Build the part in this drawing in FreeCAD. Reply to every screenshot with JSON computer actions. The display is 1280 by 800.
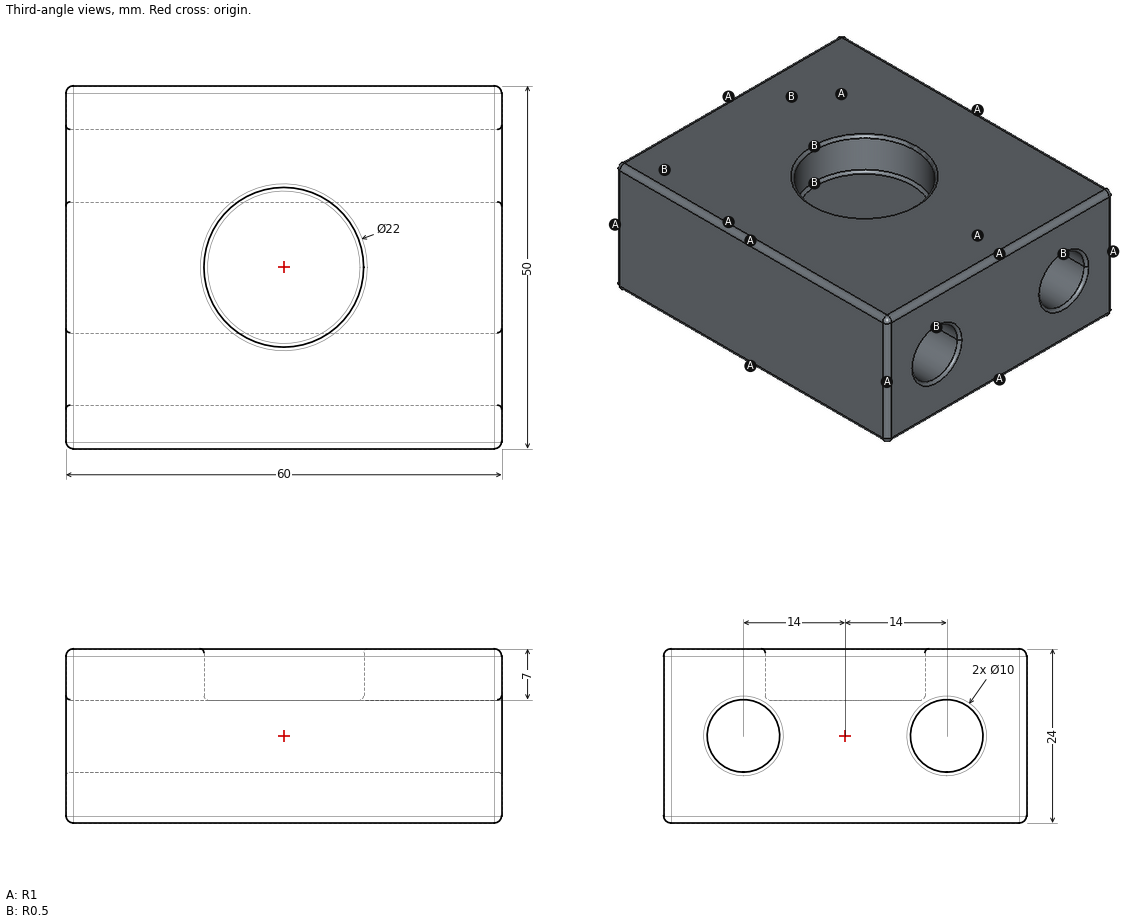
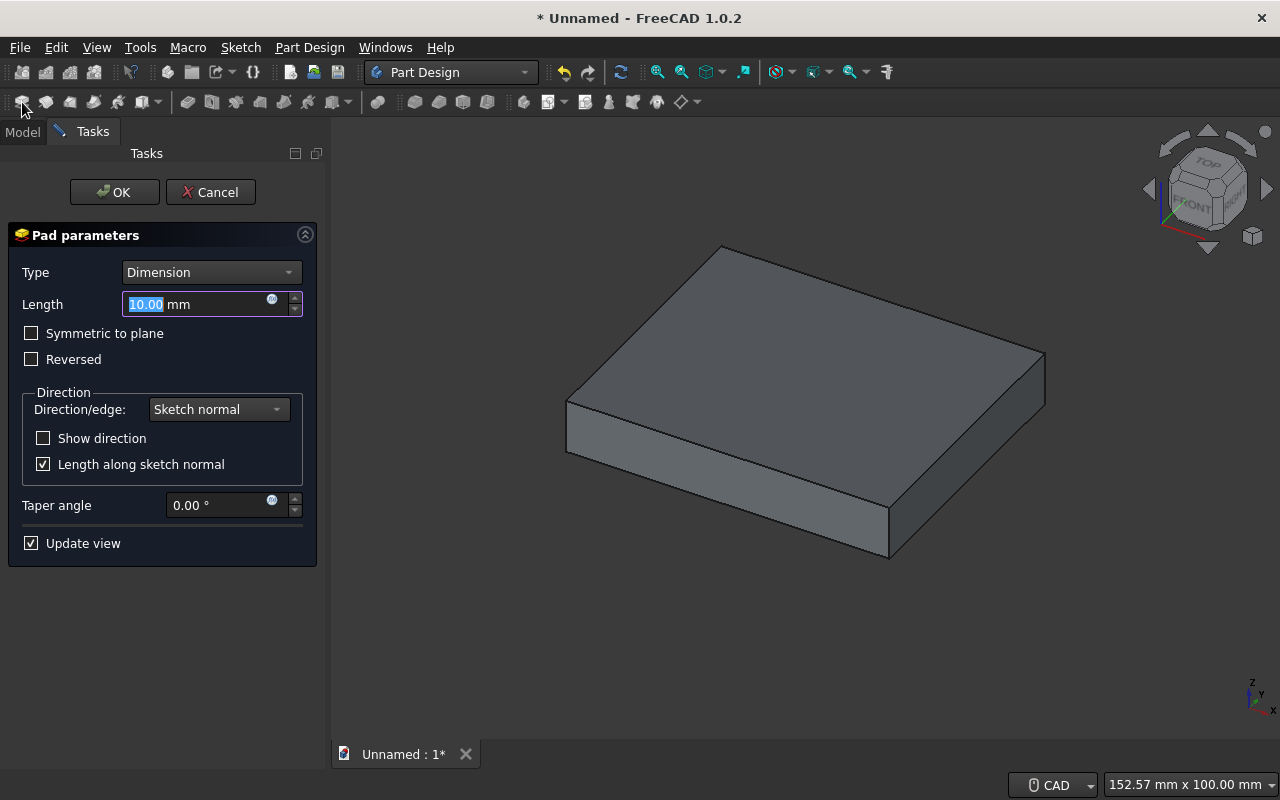
{"action": "type", "text": "24"}
{"action": "key", "text": "Tab"}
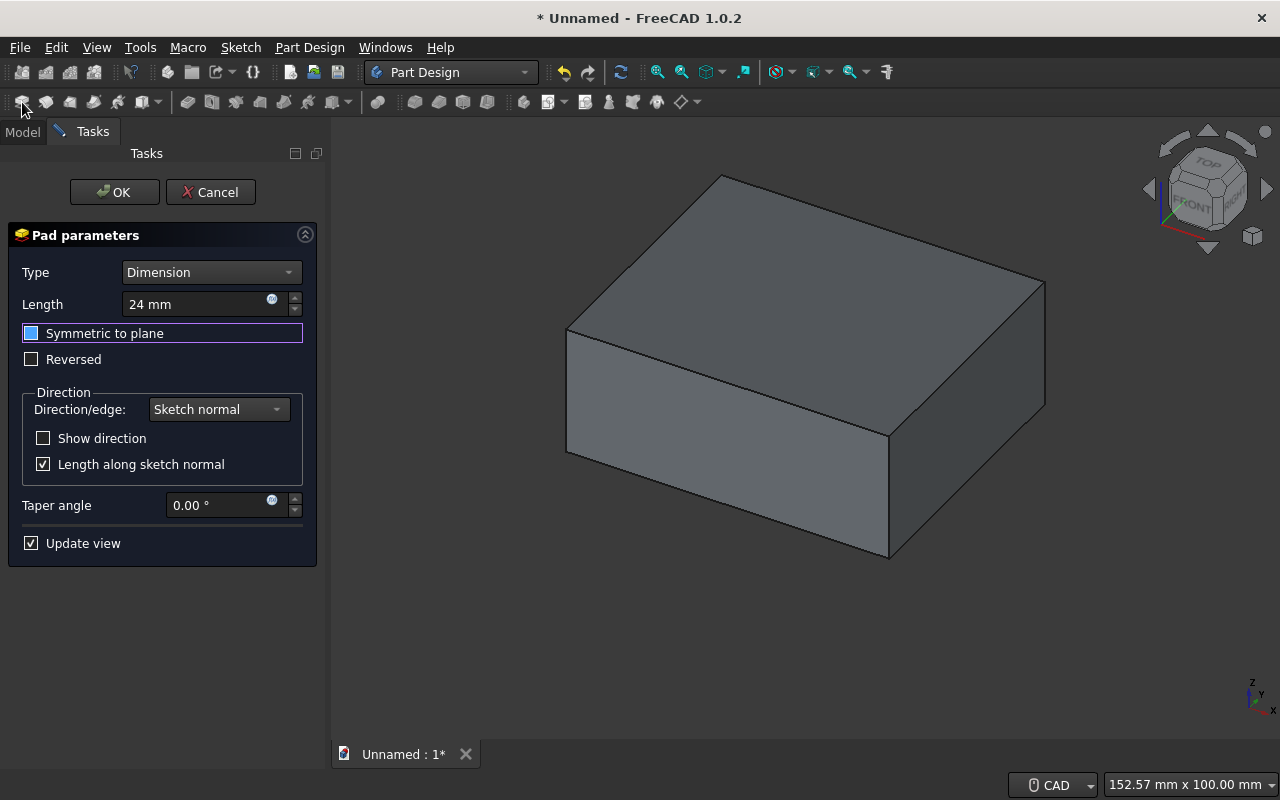
{"action": "left_click", "coordinate": [30, 333]}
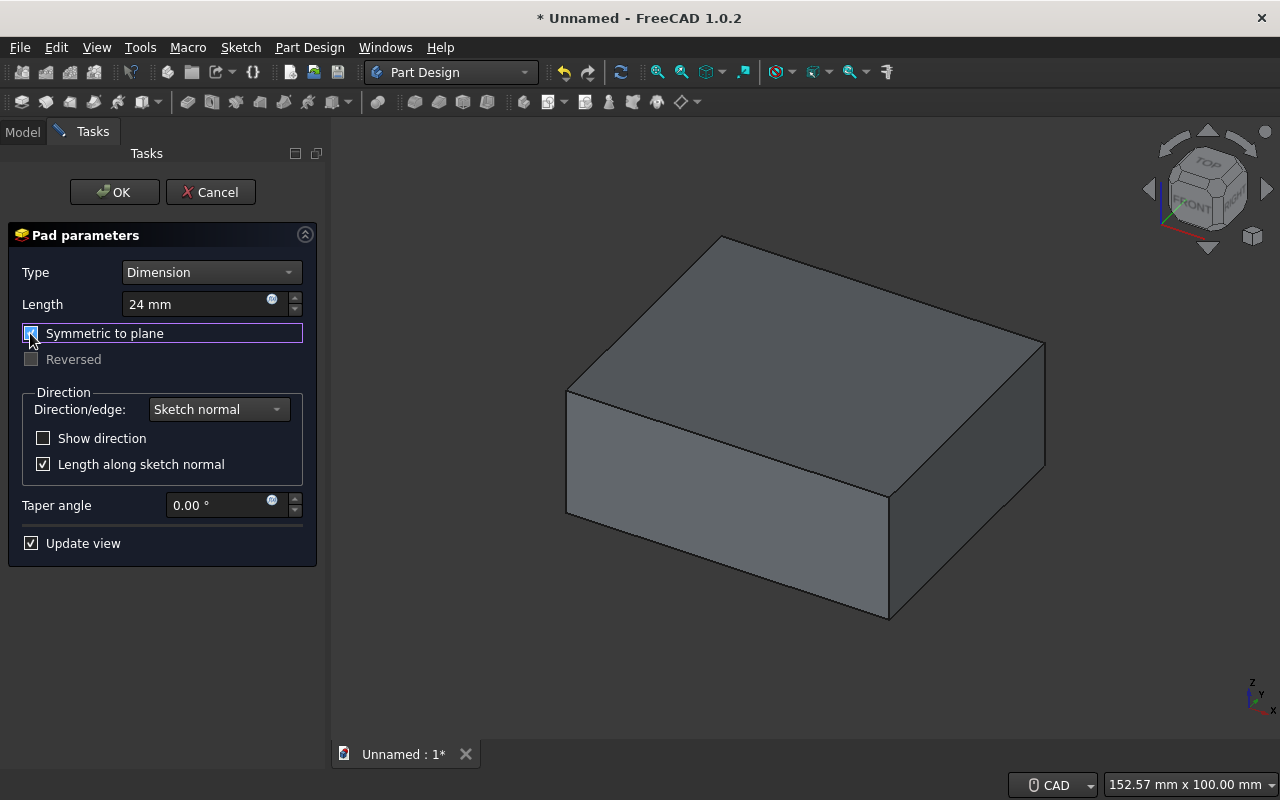
{"action": "left_click", "coordinate": [115, 192]}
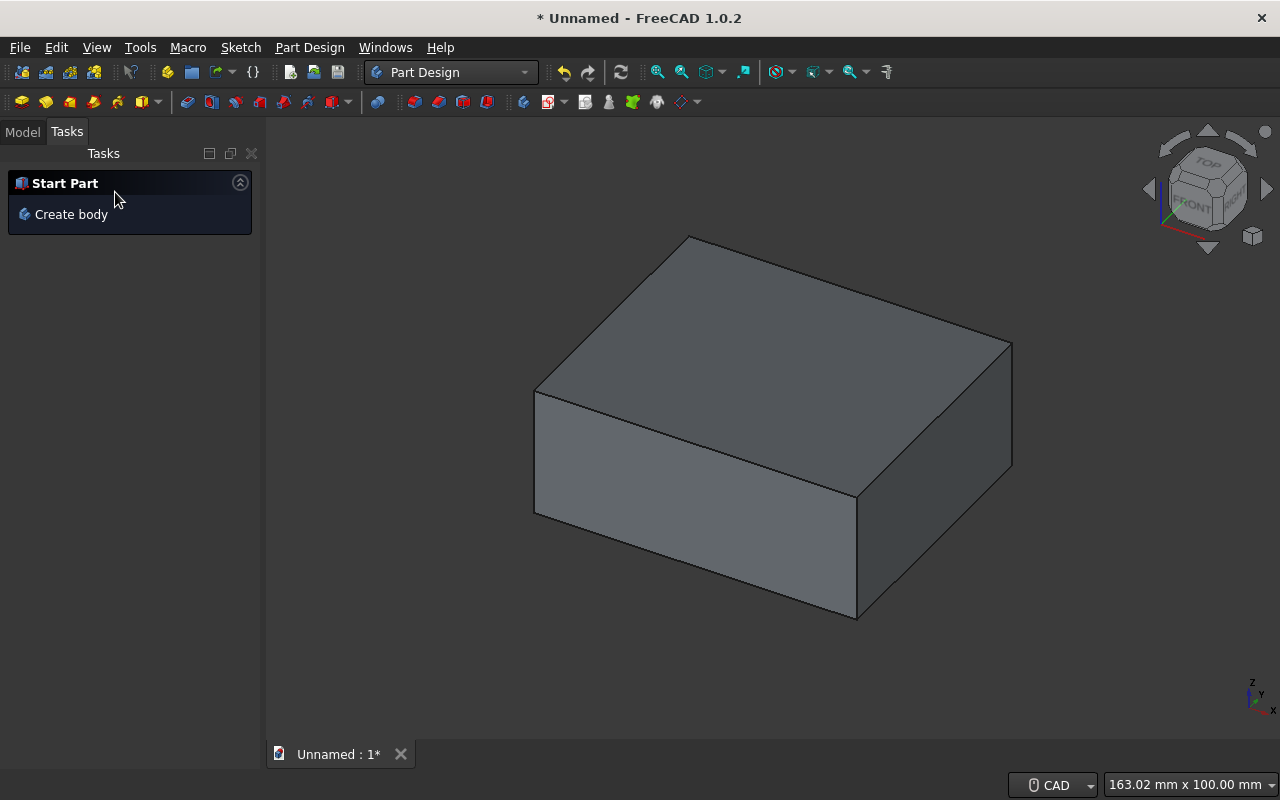
{"action": "left_click", "coordinate": [773, 366]}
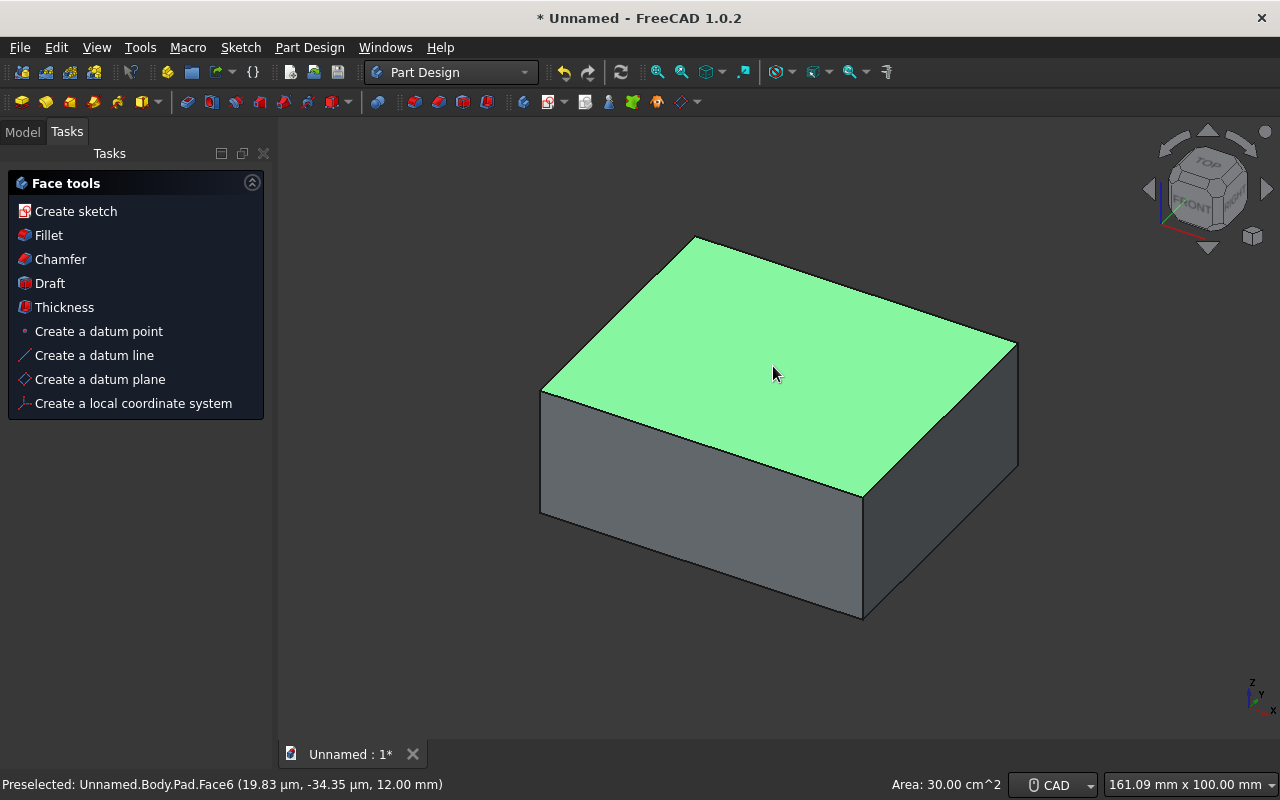
{"action": "left_click", "coordinate": [548, 102]}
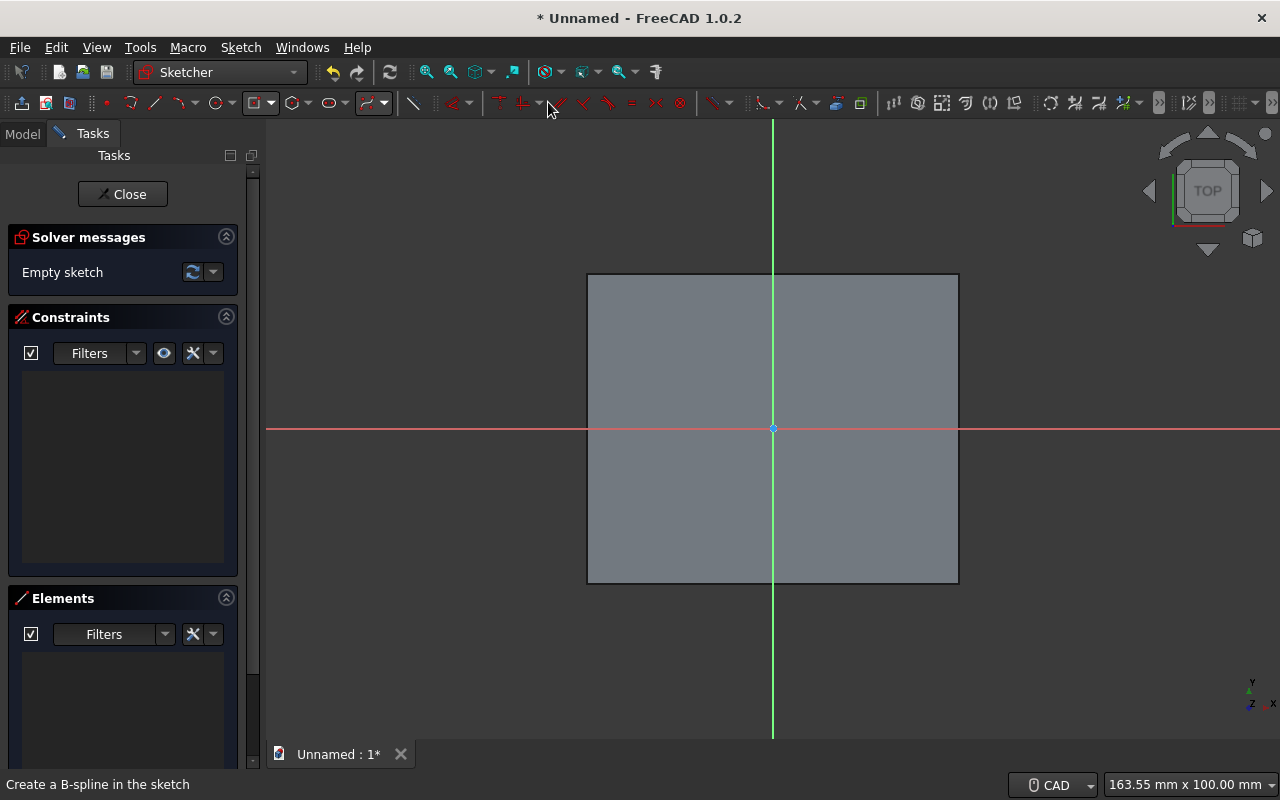
{"action": "scroll", "coordinate": [813, 429], "scroll_direction": "up", "scroll_amount": 5}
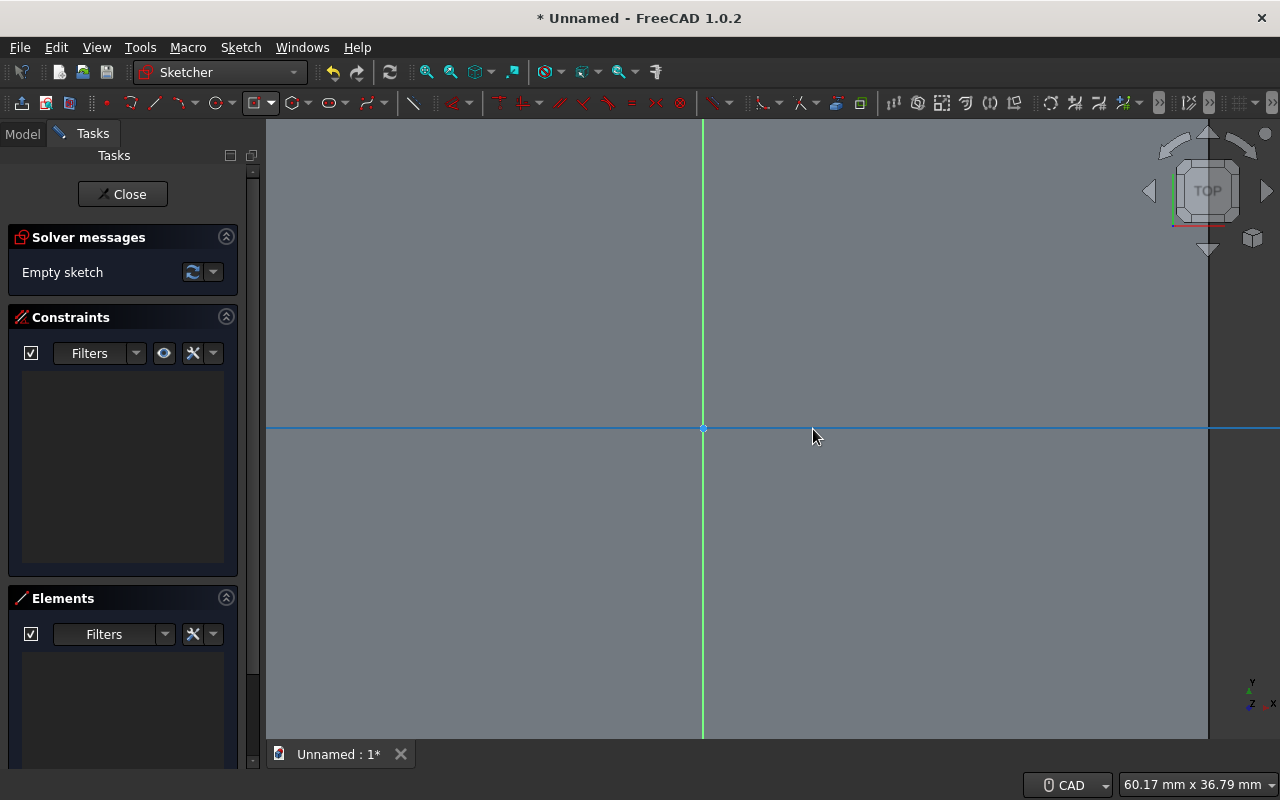
{"action": "left_click", "coordinate": [216, 104]}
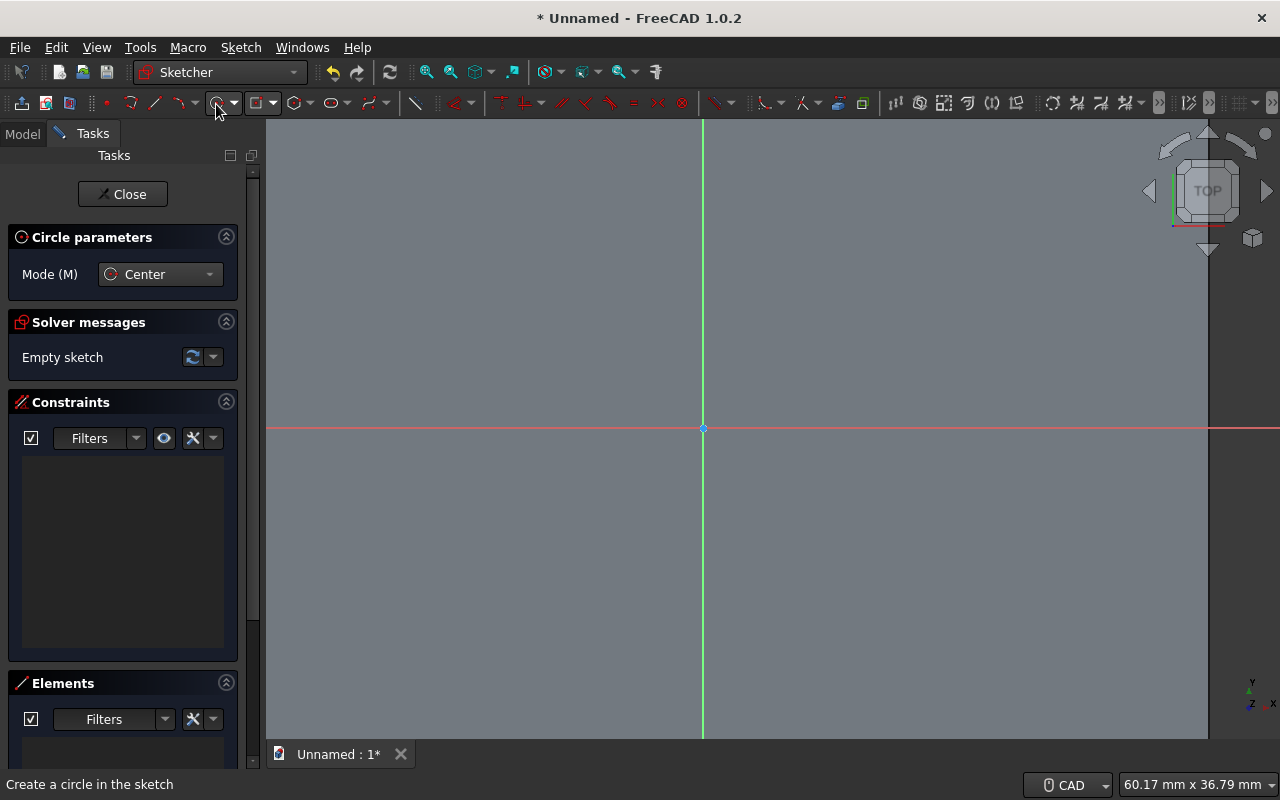
{"action": "left_click", "coordinate": [703, 428]}
{"action": "mouse_move", "coordinate": [834, 297]}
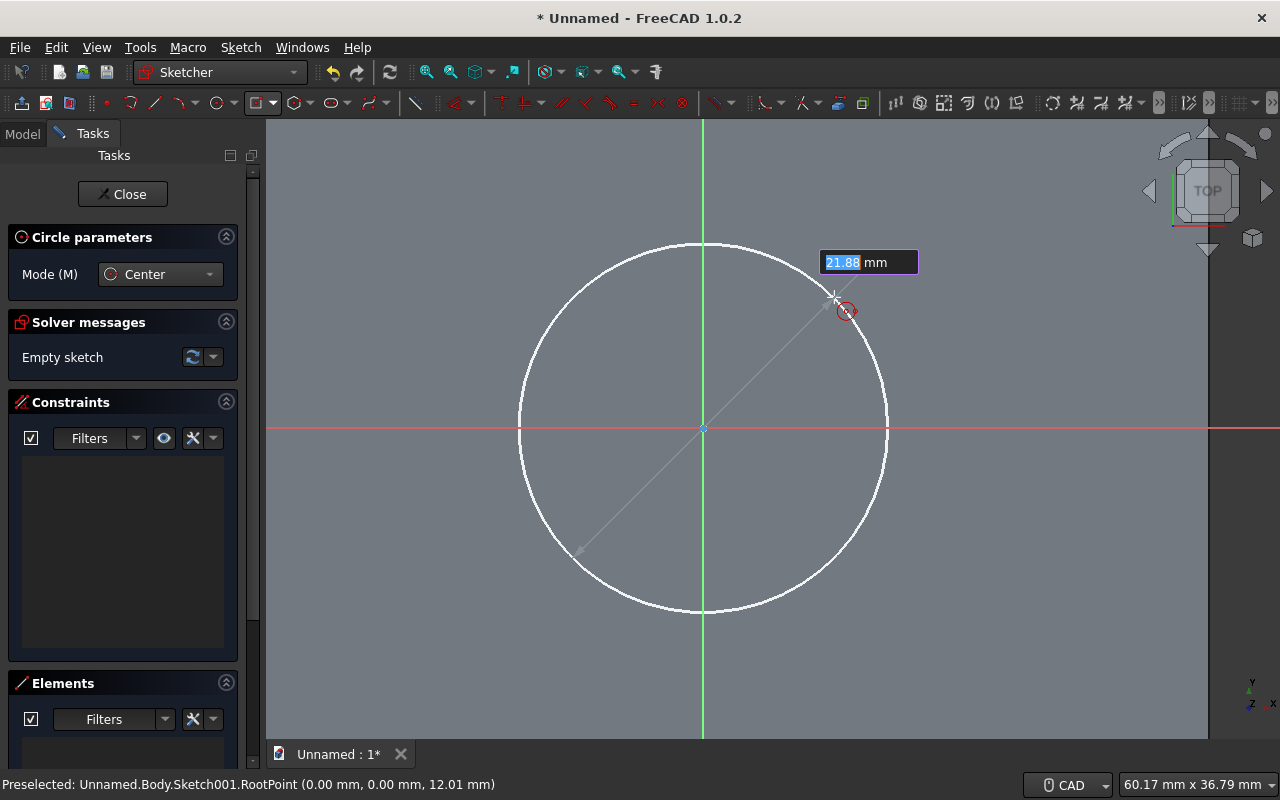
{"action": "type", "text": "22"}
{"action": "key", "text": "Return"}
{"action": "key", "text": "Escape"}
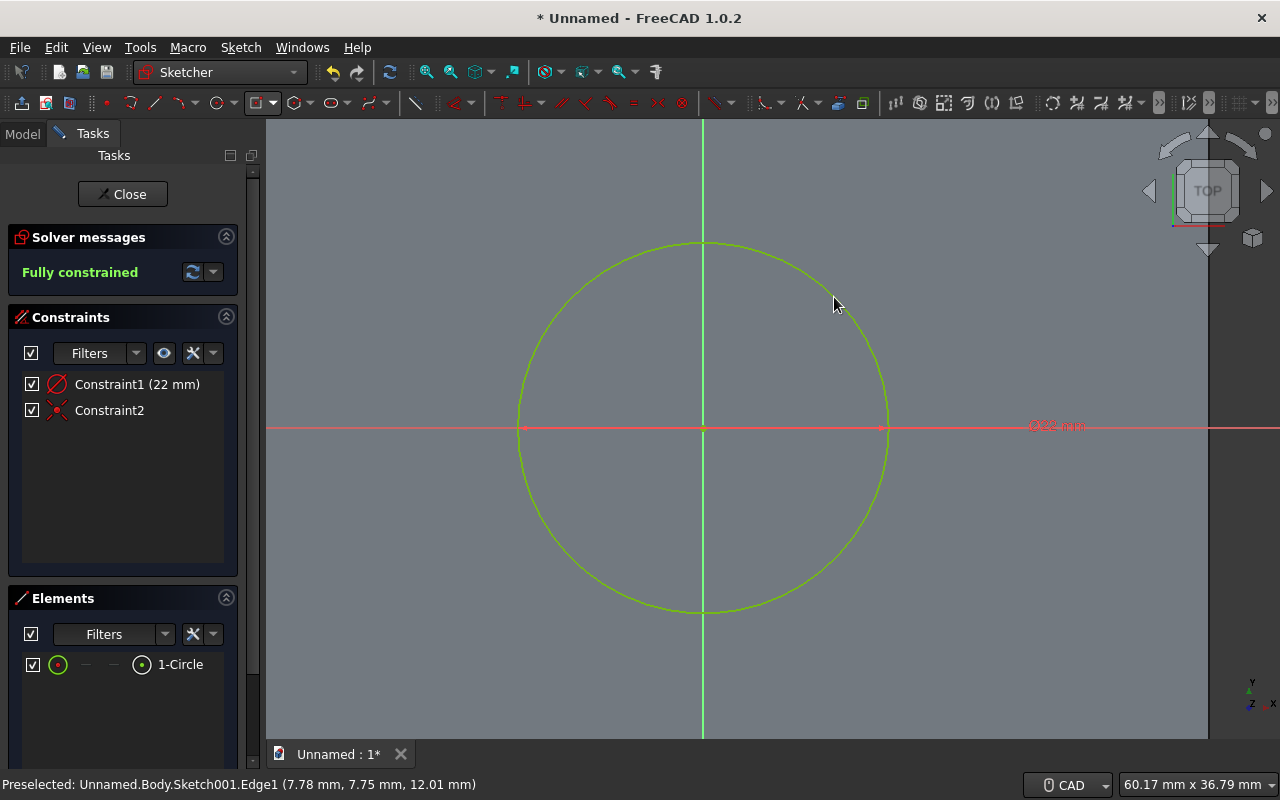
{"action": "left_click", "coordinate": [123, 194]}